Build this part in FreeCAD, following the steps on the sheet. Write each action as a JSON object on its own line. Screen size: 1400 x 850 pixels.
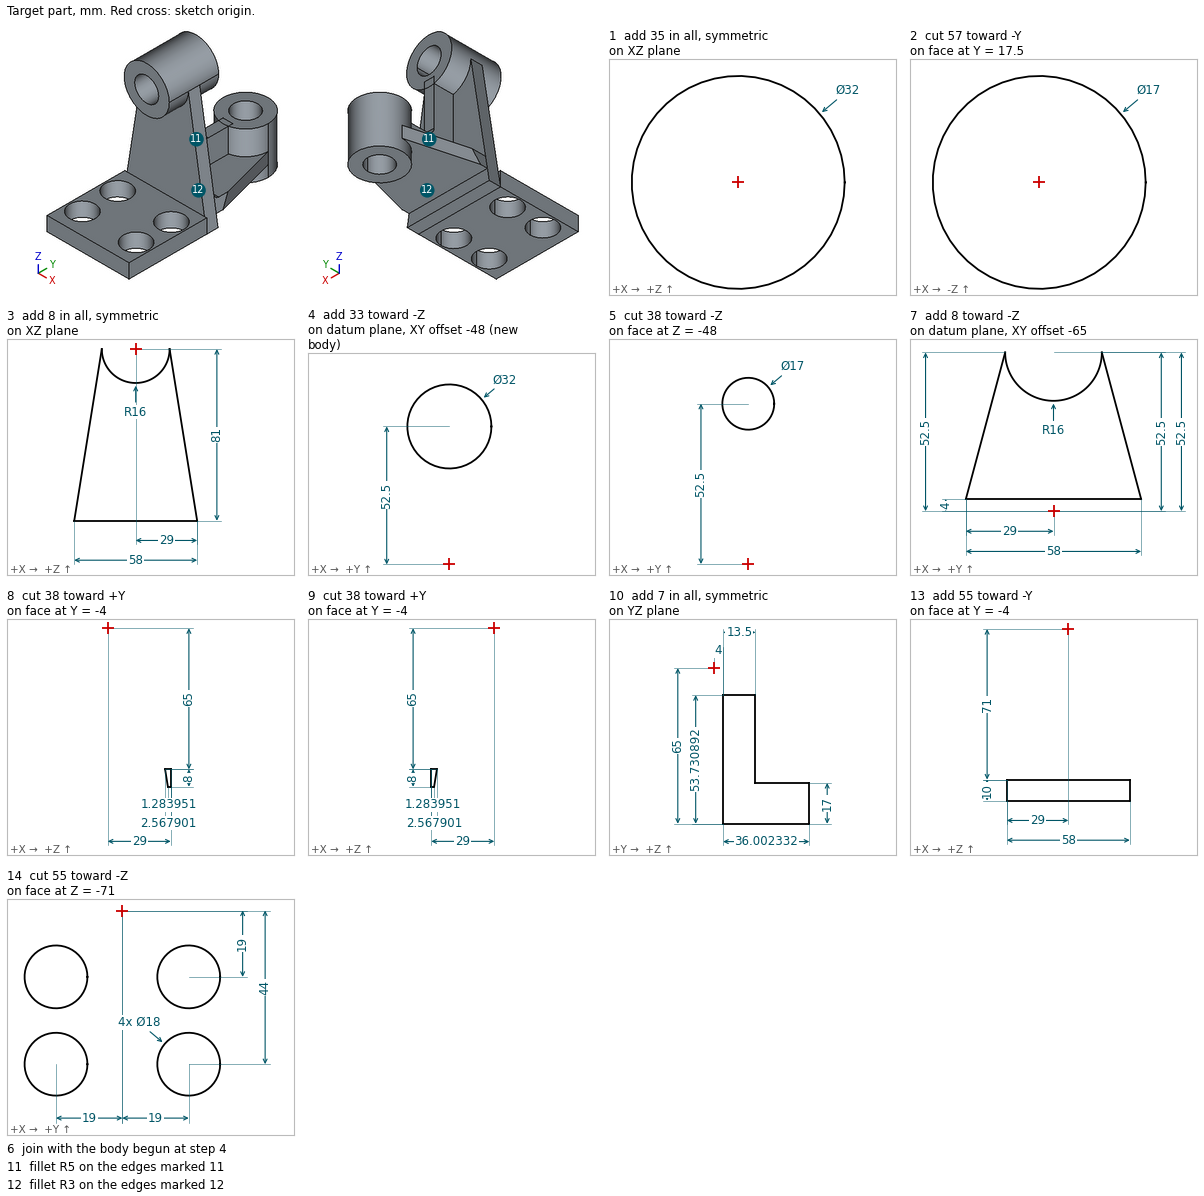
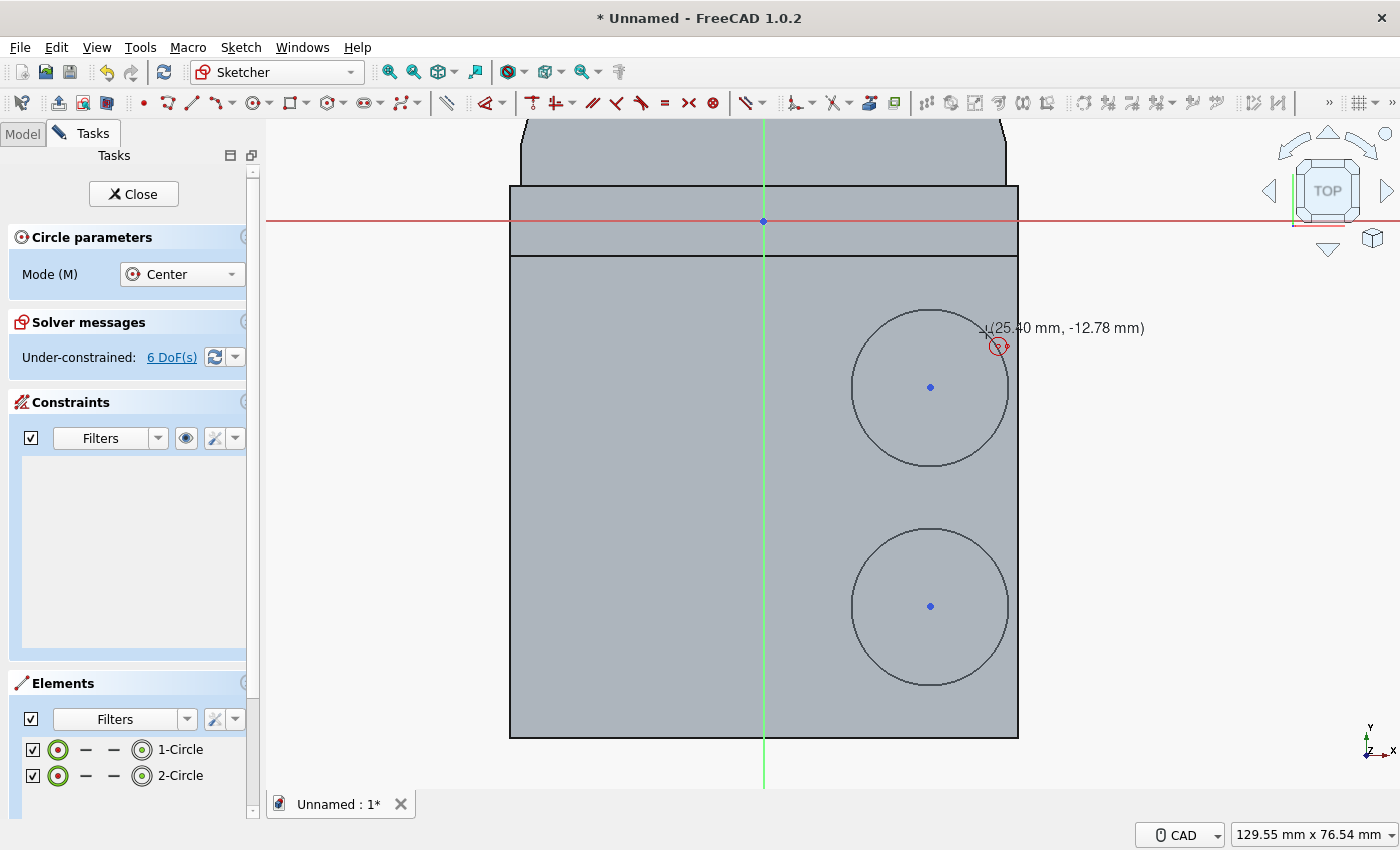
{"action": "left_click", "coordinate": [597, 606]}
{"action": "left_click", "coordinate": [653, 551]}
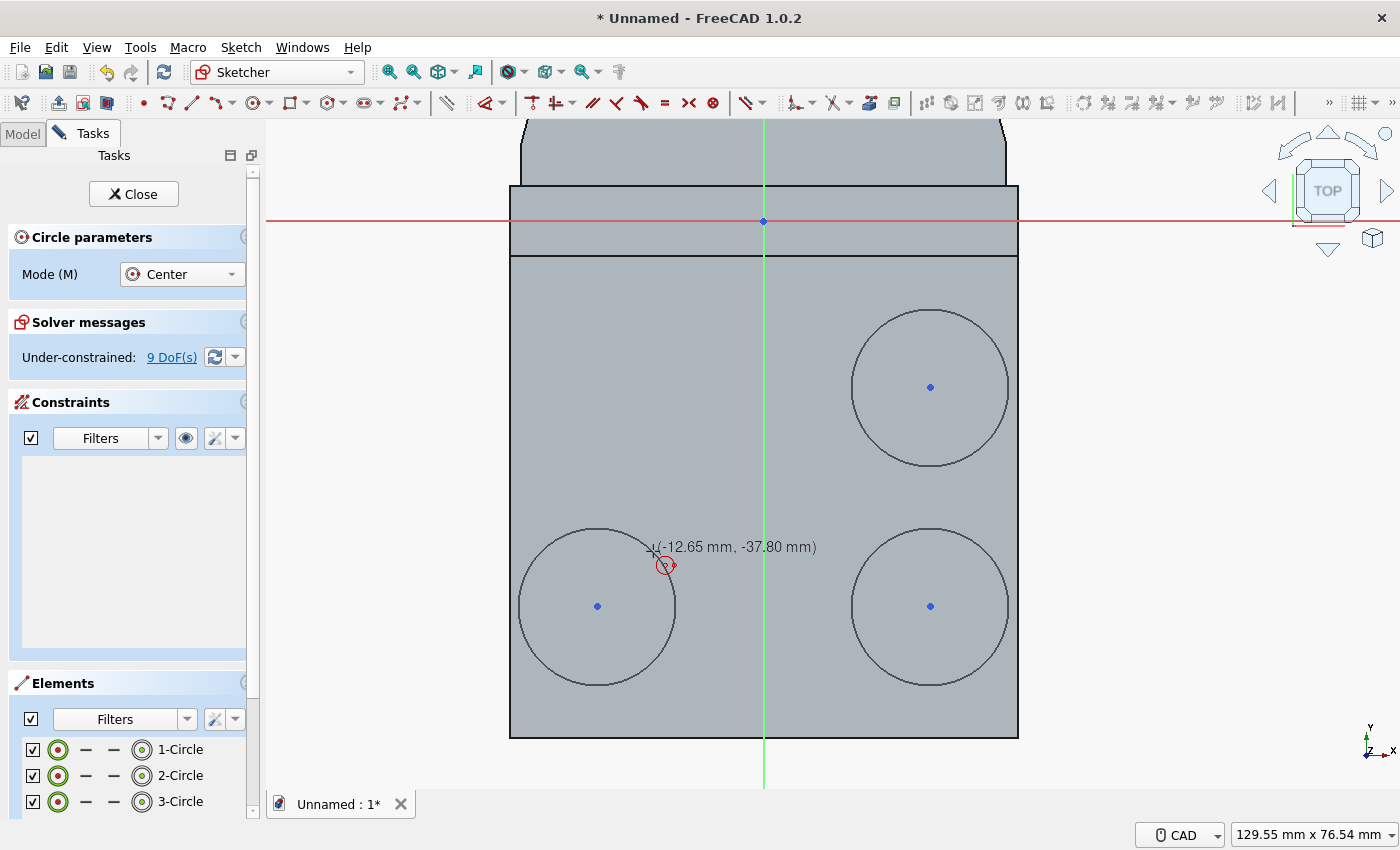
{"action": "left_click", "coordinate": [597, 387]}
{"action": "left_click", "coordinate": [653, 332]}
{"action": "key", "text": "Escape"}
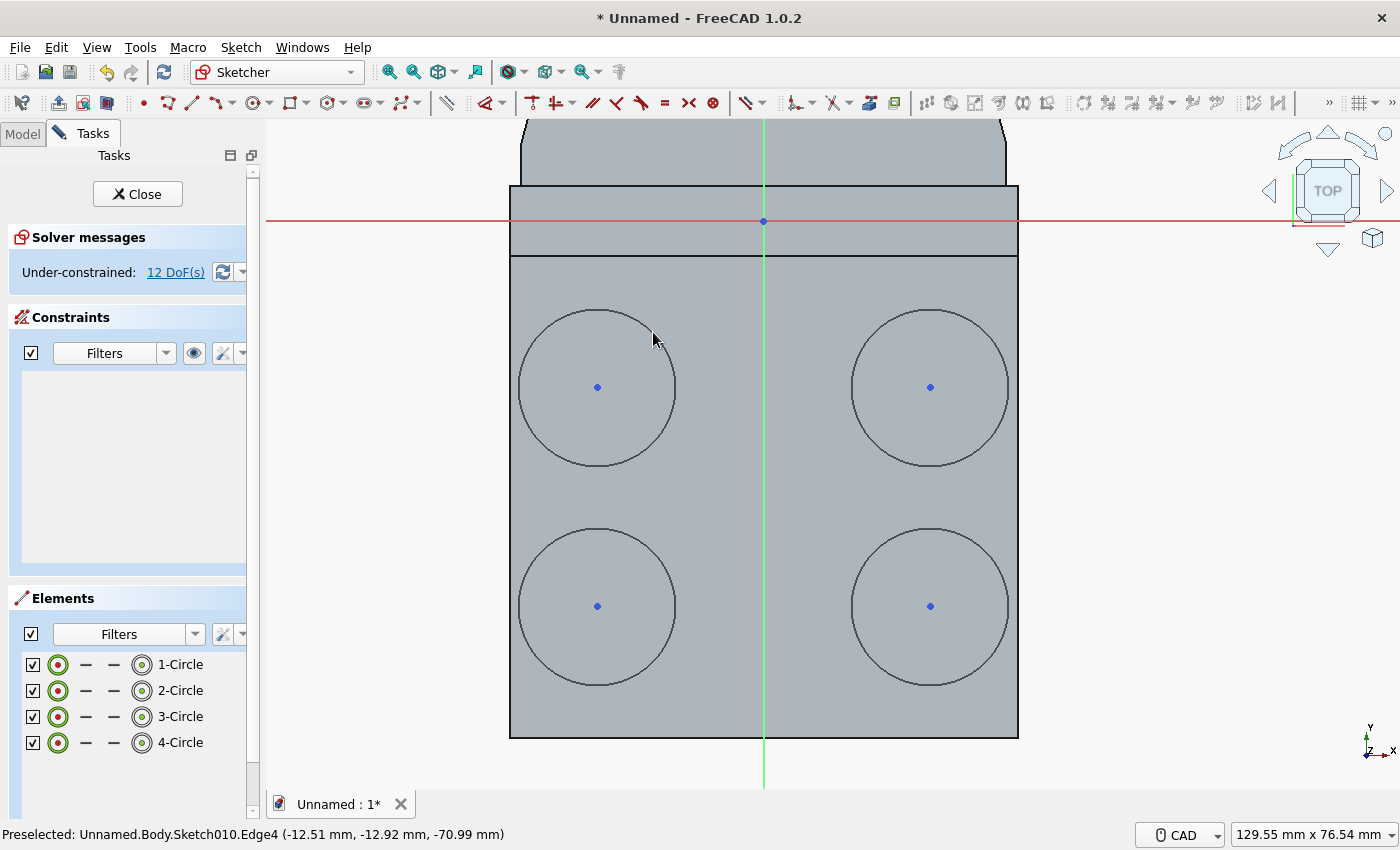
{"action": "left_click", "coordinate": [985, 551]}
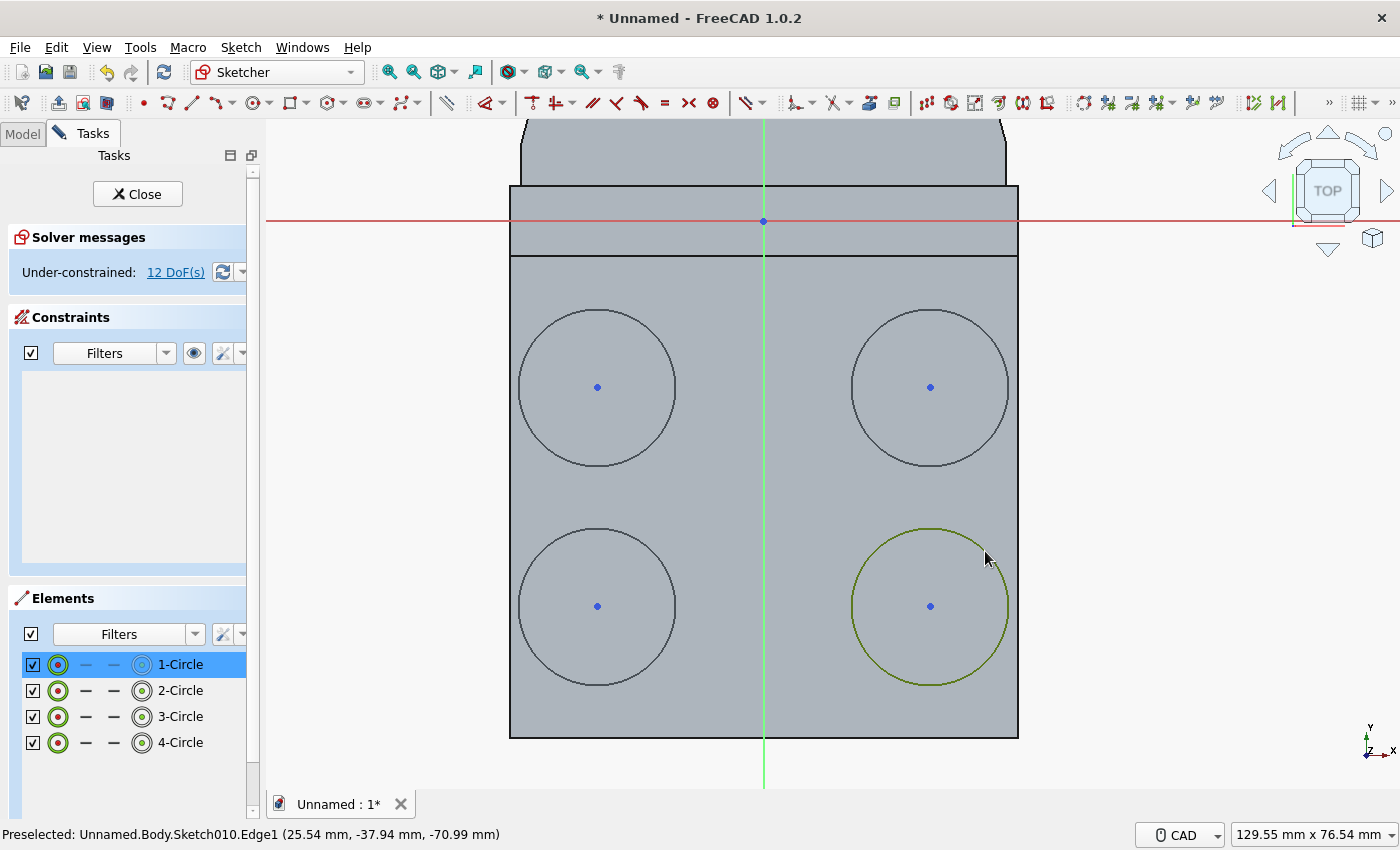
{"action": "left_click", "coordinate": [985, 332]}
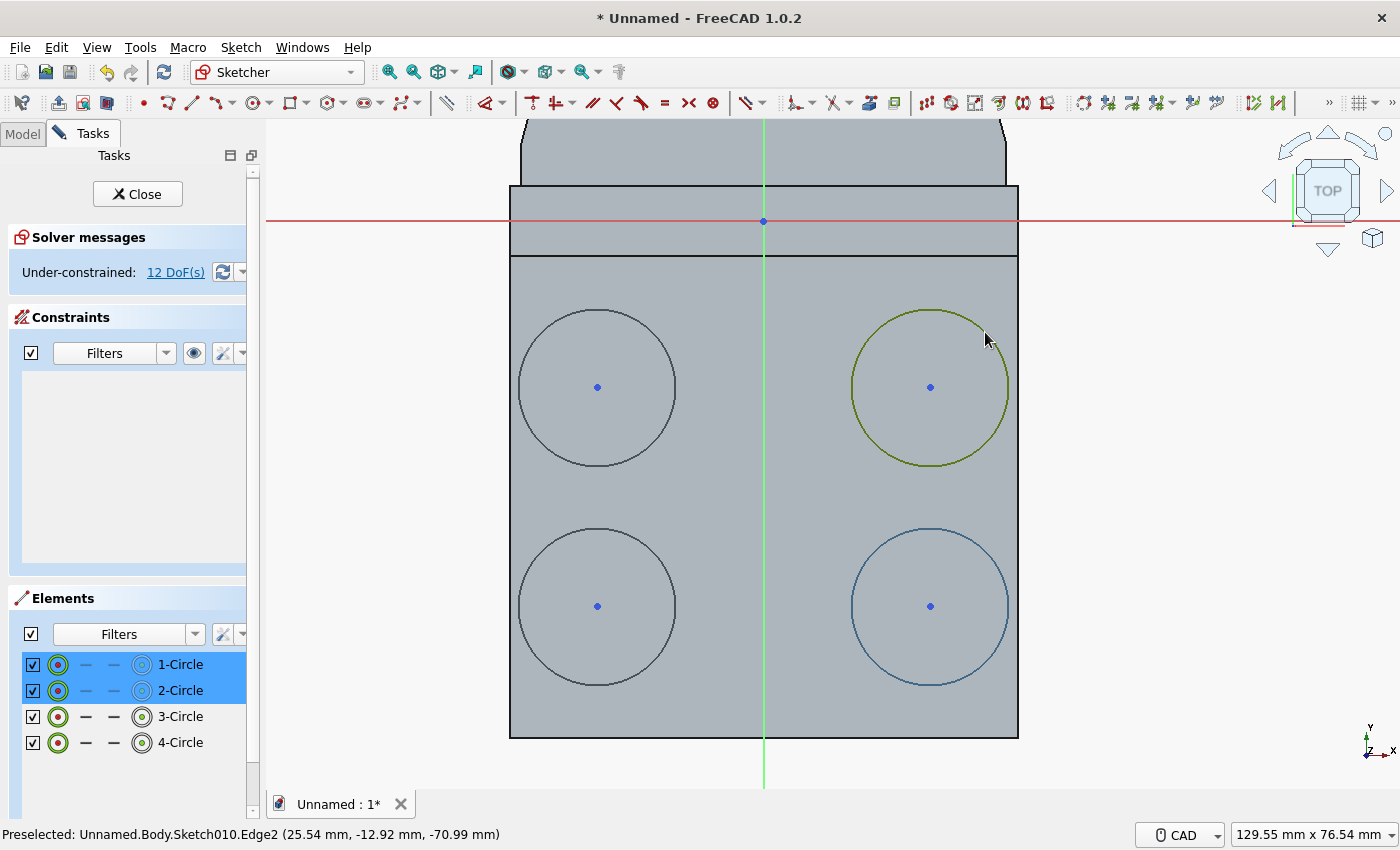
{"action": "left_click", "coordinate": [652, 551]}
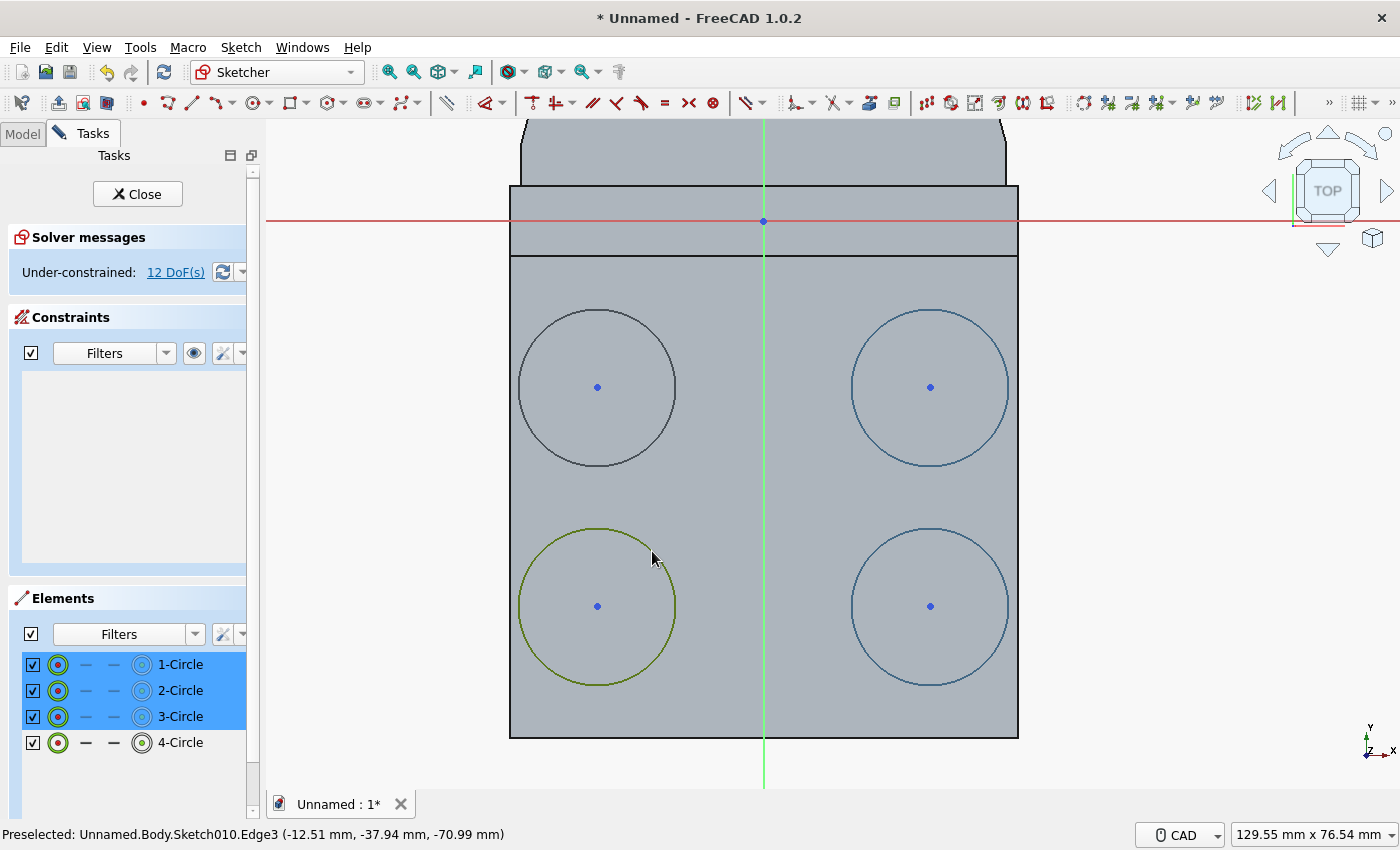
{"action": "left_click", "coordinate": [652, 332]}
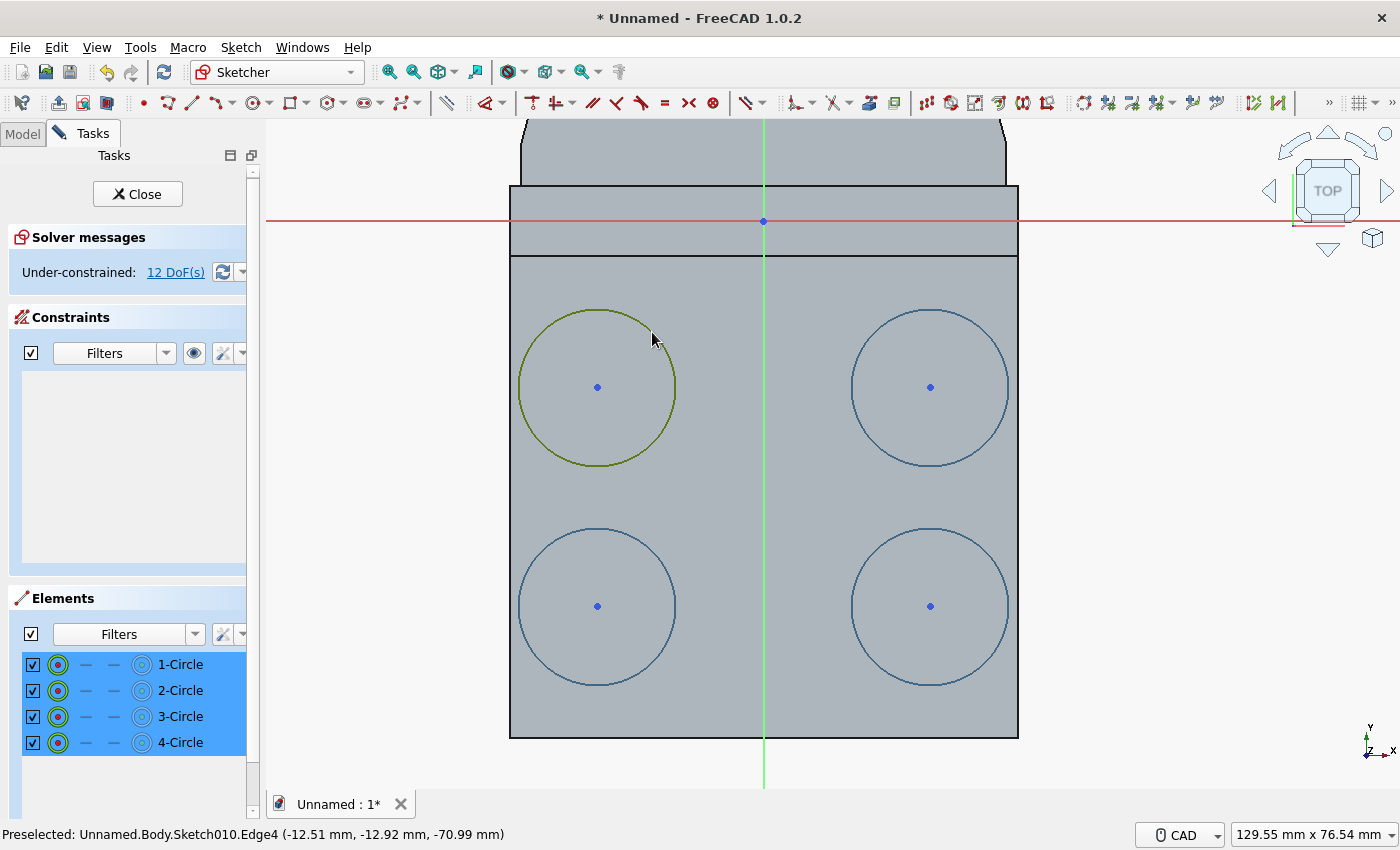
{"action": "key", "text": "e"}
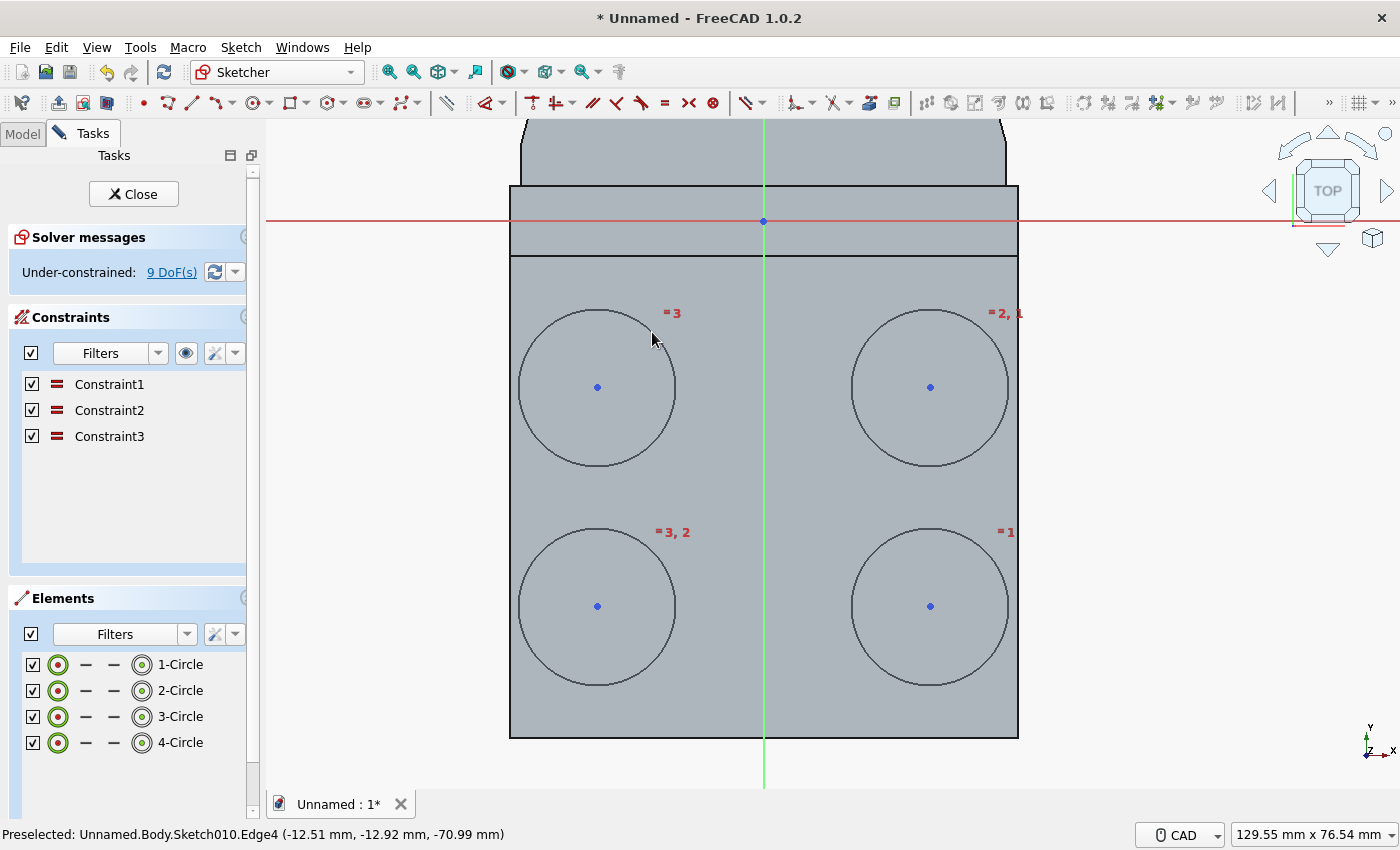
{"action": "left_click", "coordinate": [930, 607]}